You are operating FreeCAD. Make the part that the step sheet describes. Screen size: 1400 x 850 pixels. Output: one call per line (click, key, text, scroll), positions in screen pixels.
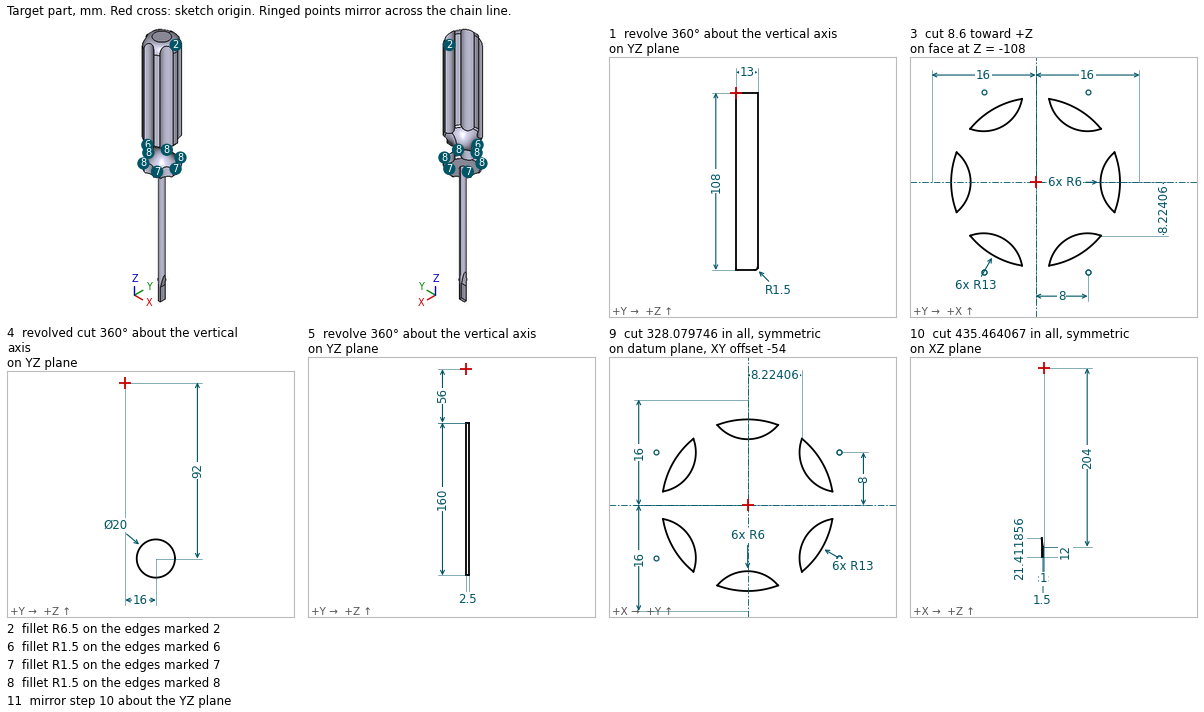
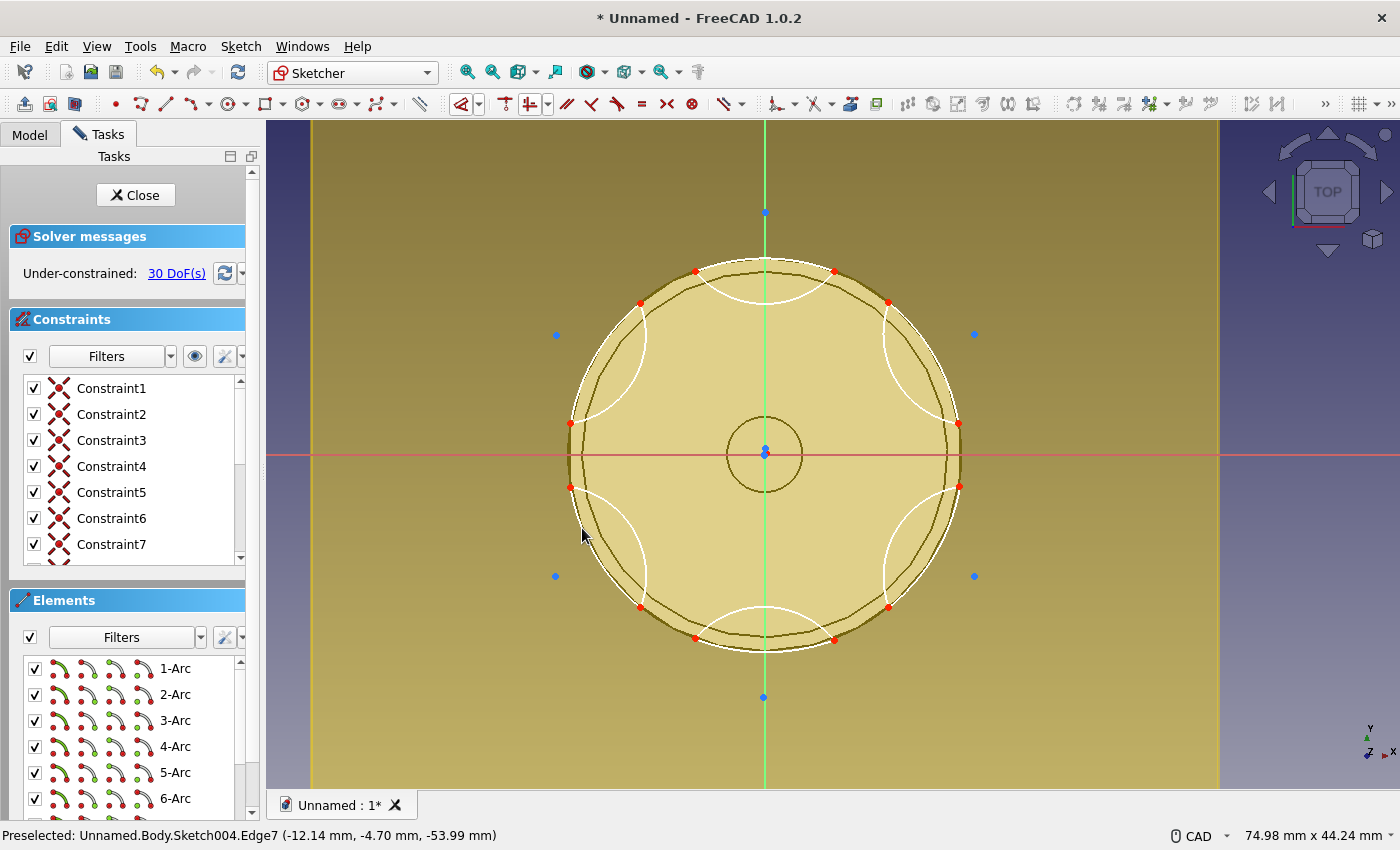
click(947, 383)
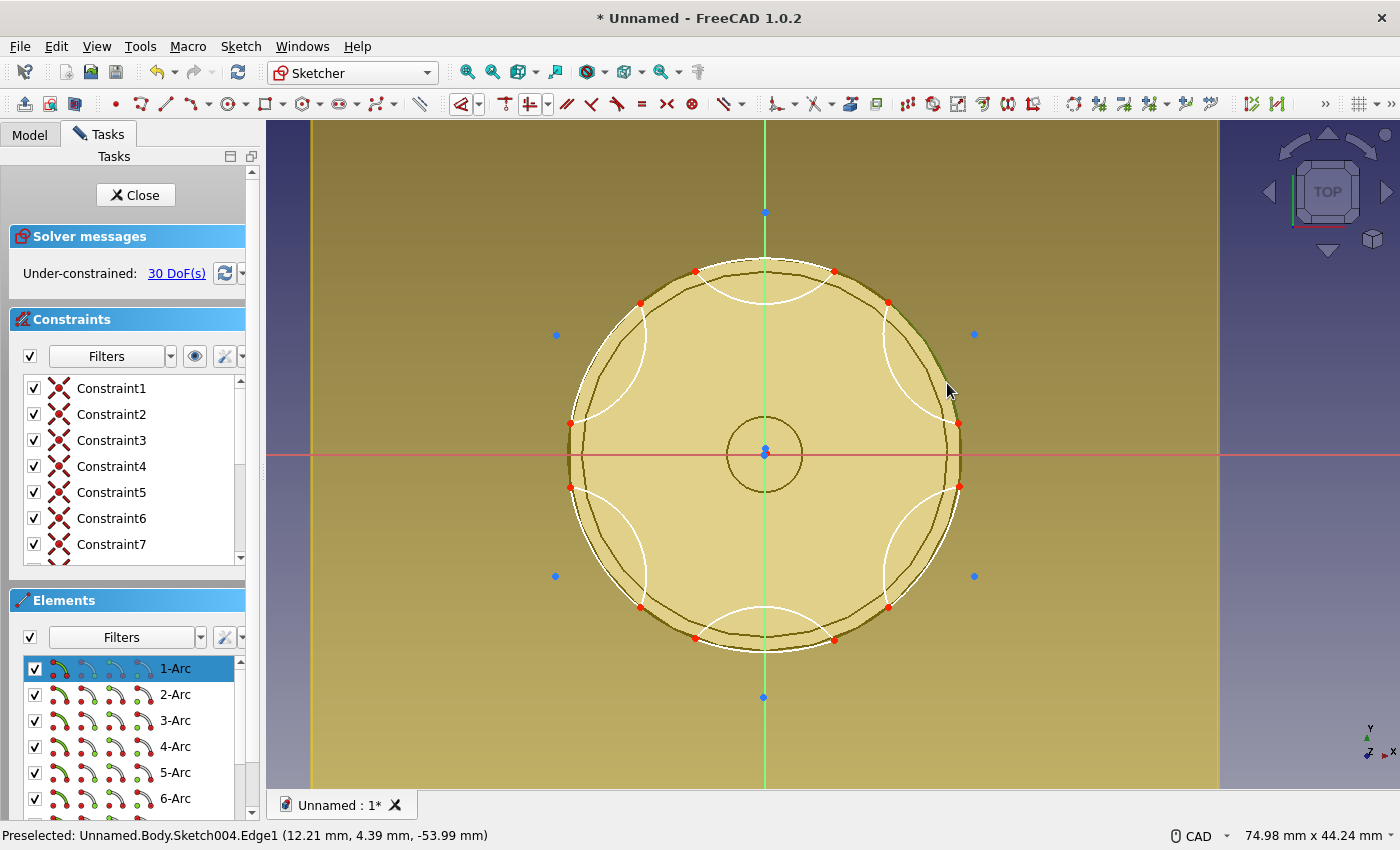
click(610, 334)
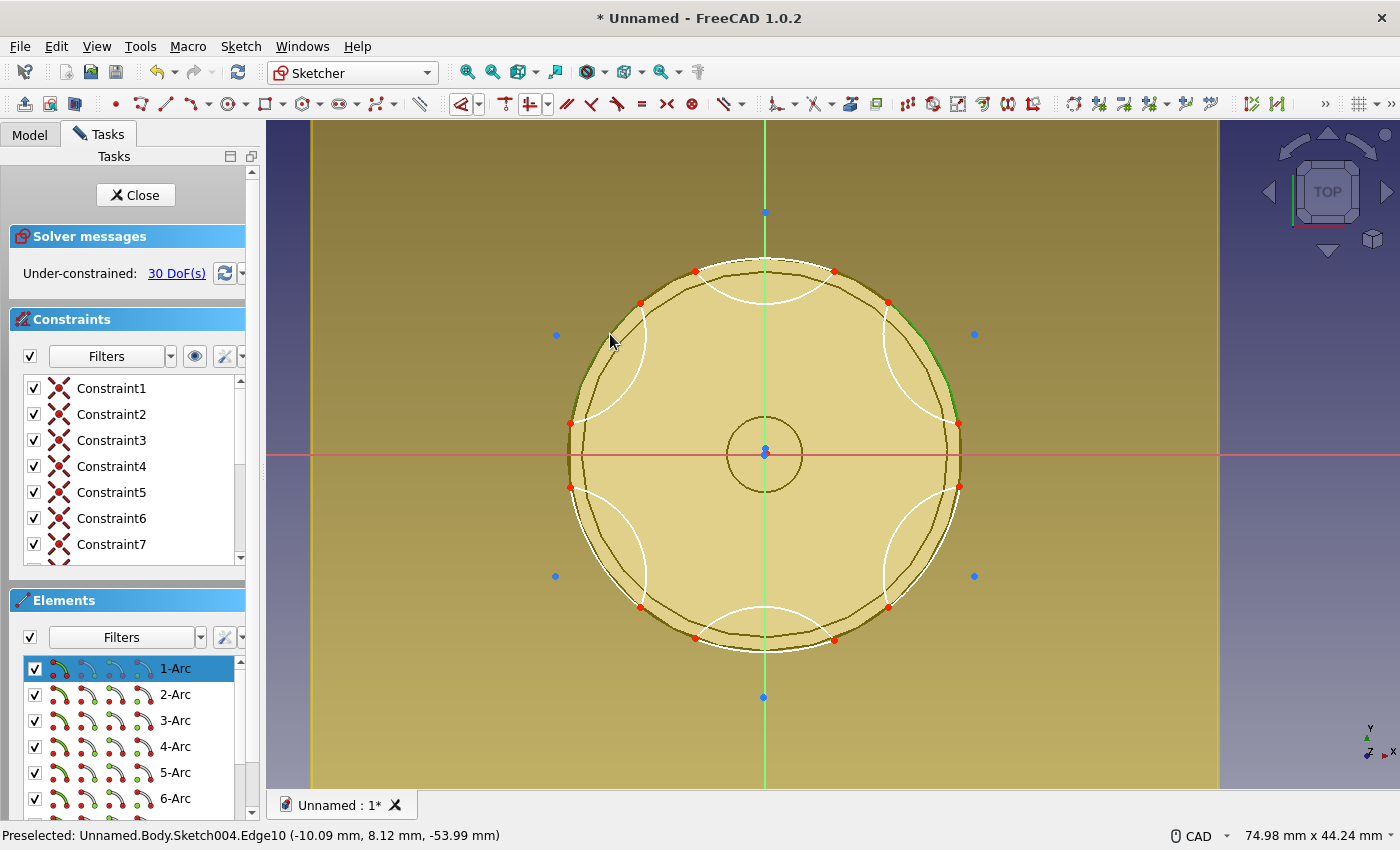
key(c)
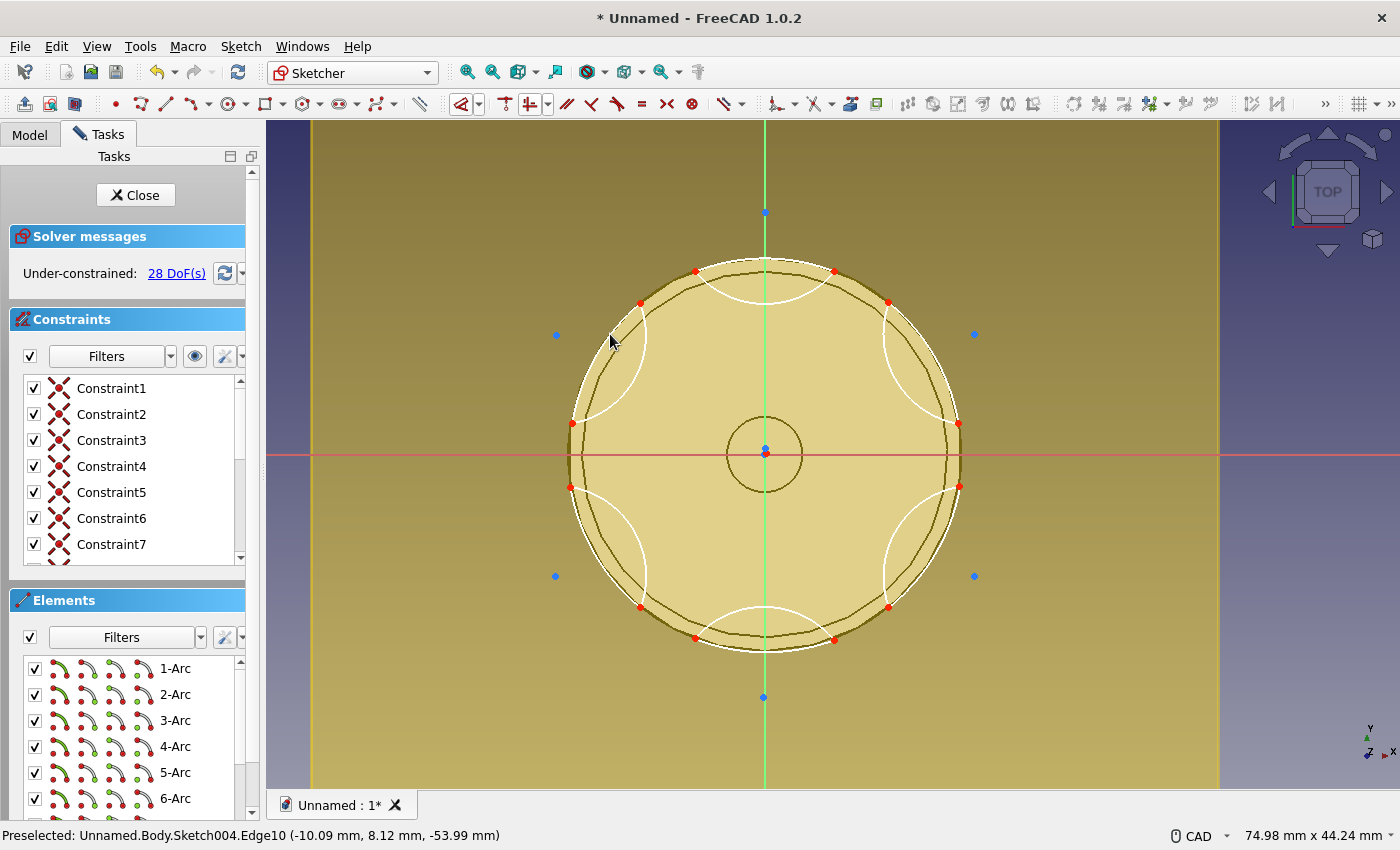
click(947, 383)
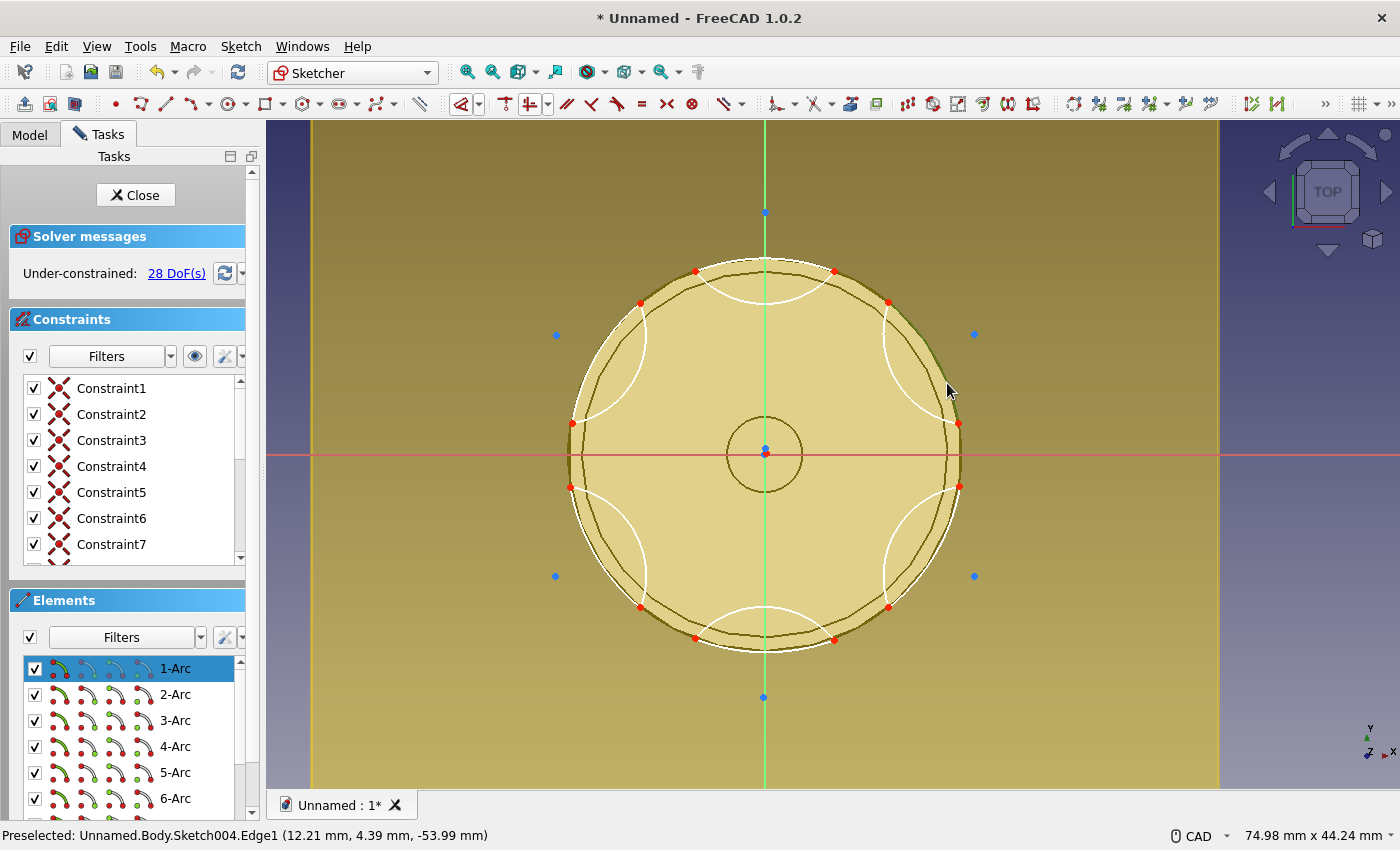
click(793, 261)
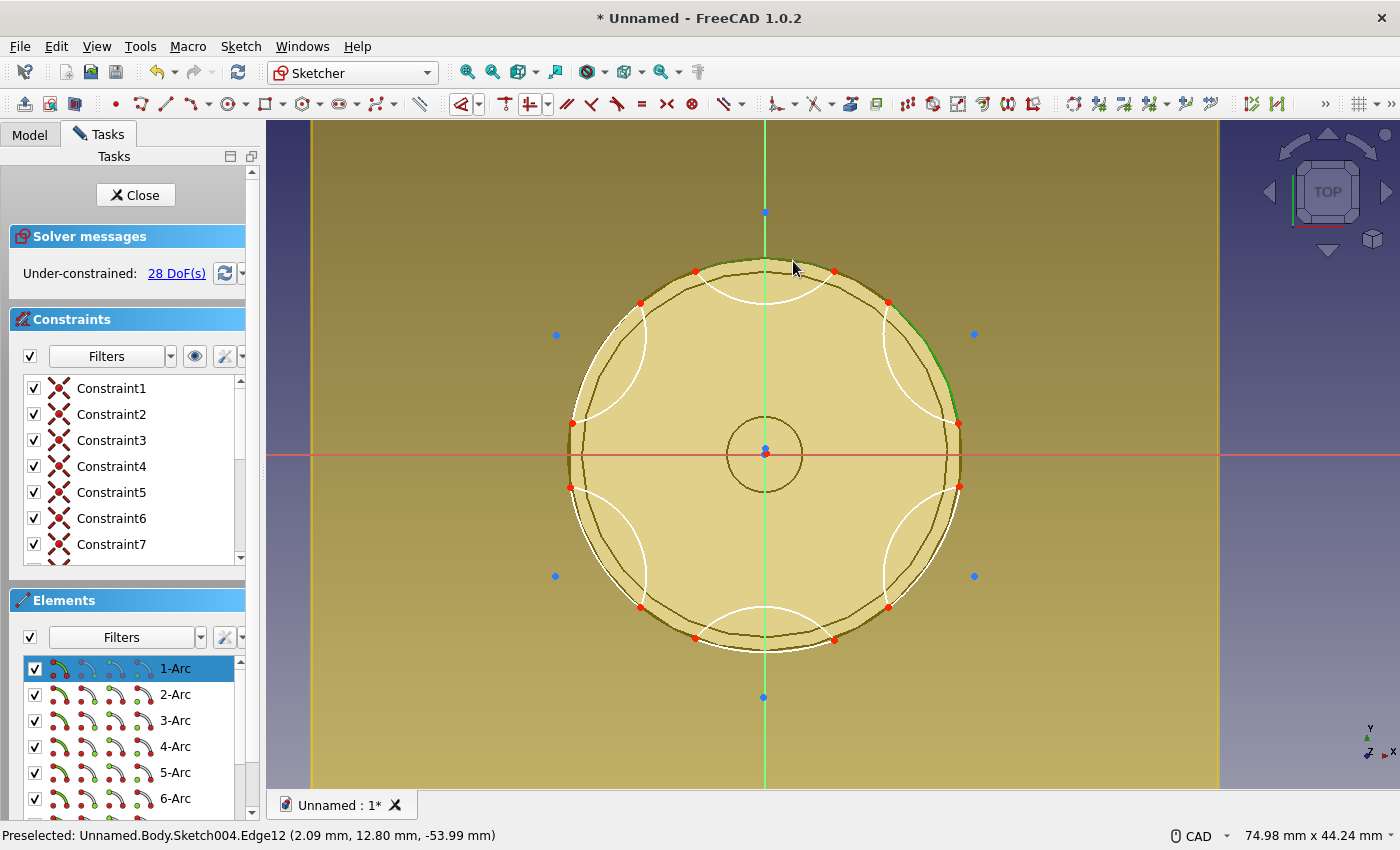
key(c)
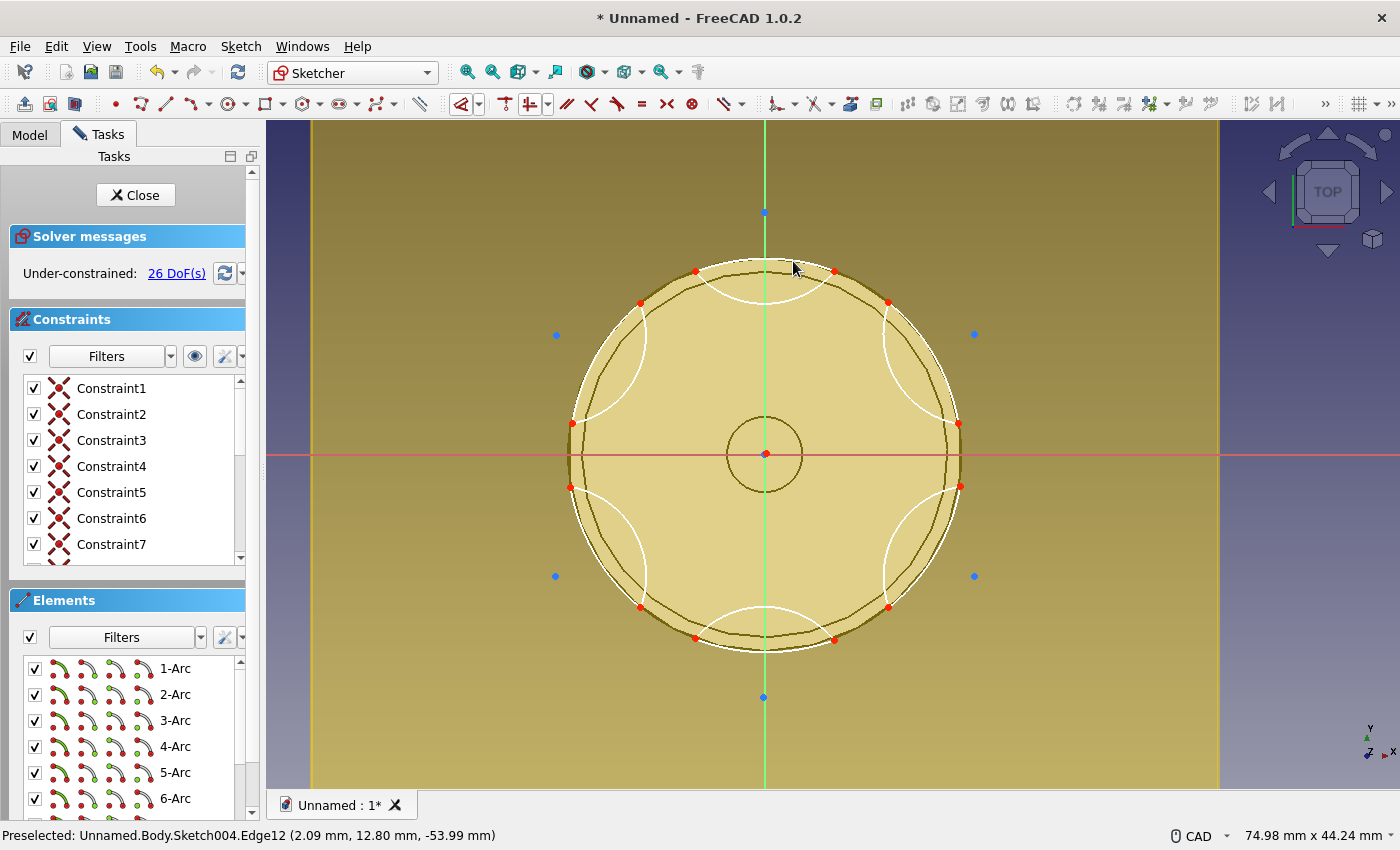
drag(755, 444, 776, 465)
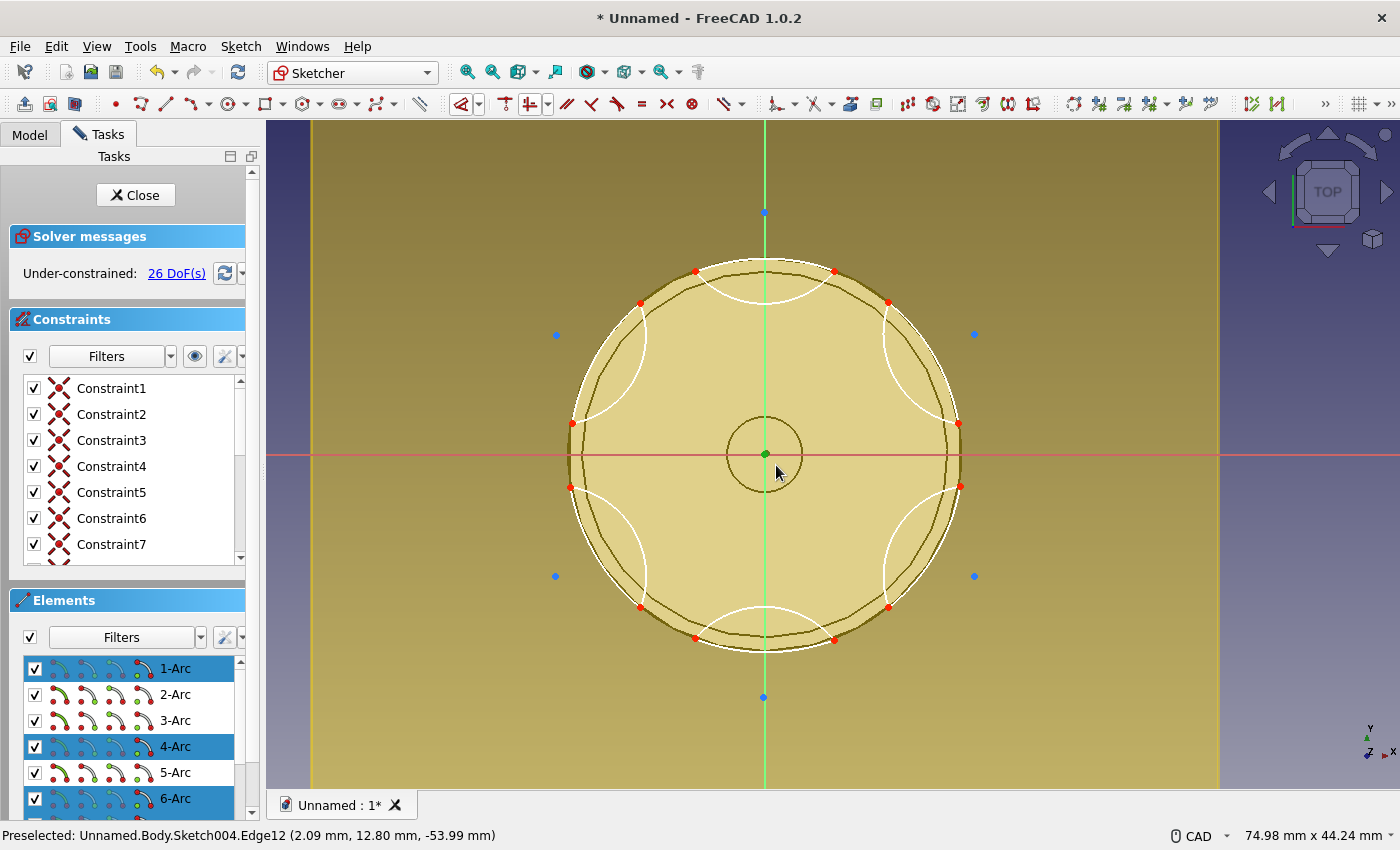
key(c)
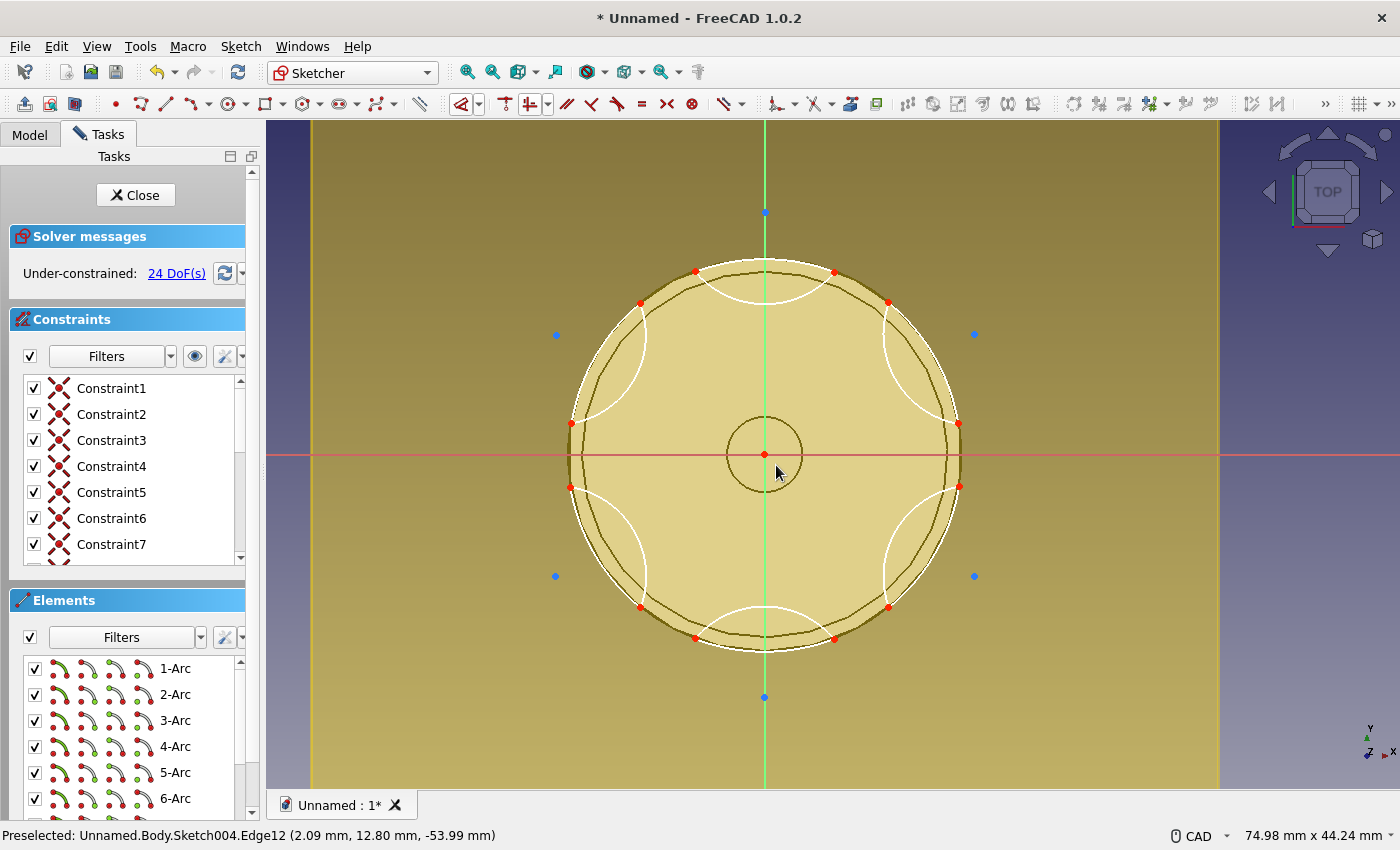
click(885, 350)